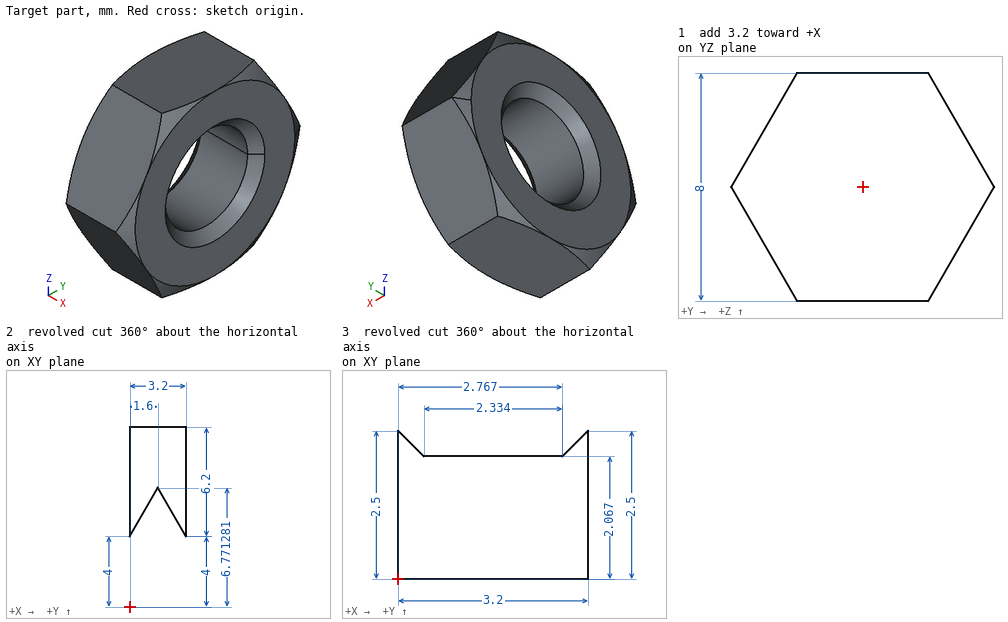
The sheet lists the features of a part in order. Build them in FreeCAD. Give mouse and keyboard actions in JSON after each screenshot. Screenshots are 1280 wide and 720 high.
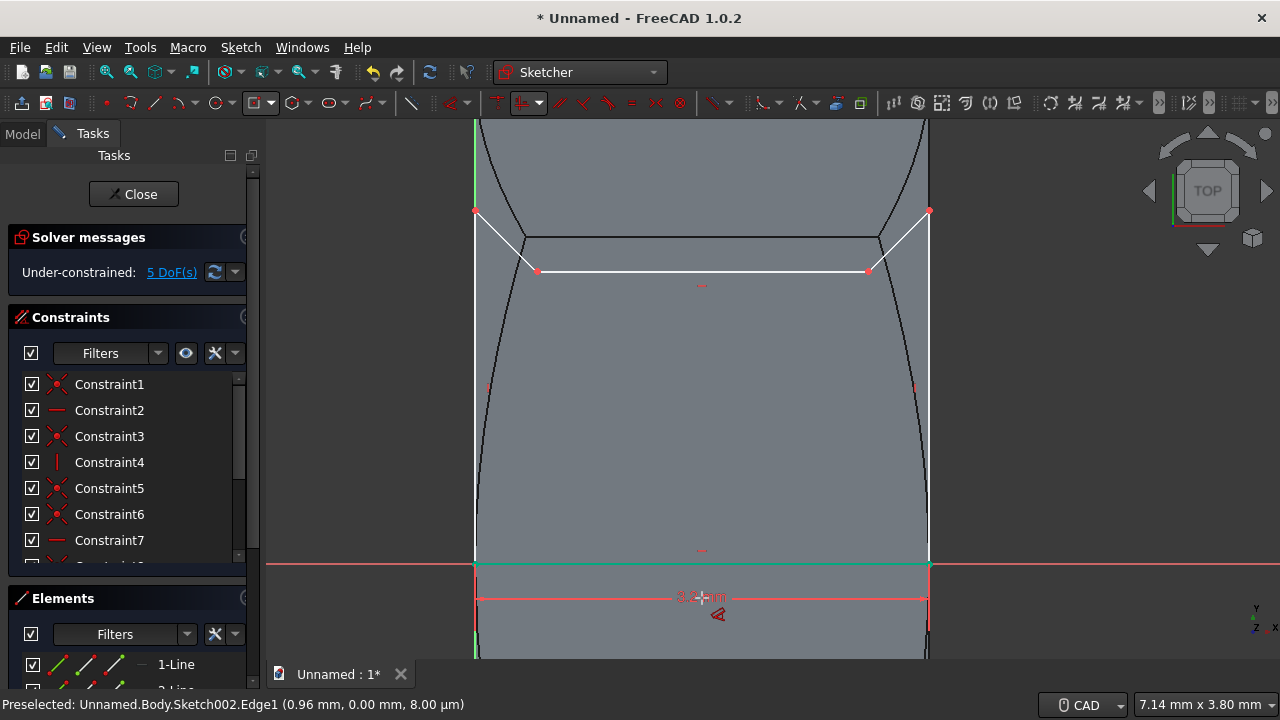
{"action": "left_click", "coordinate": [929, 458]}
{"action": "left_click", "coordinate": [963, 388]}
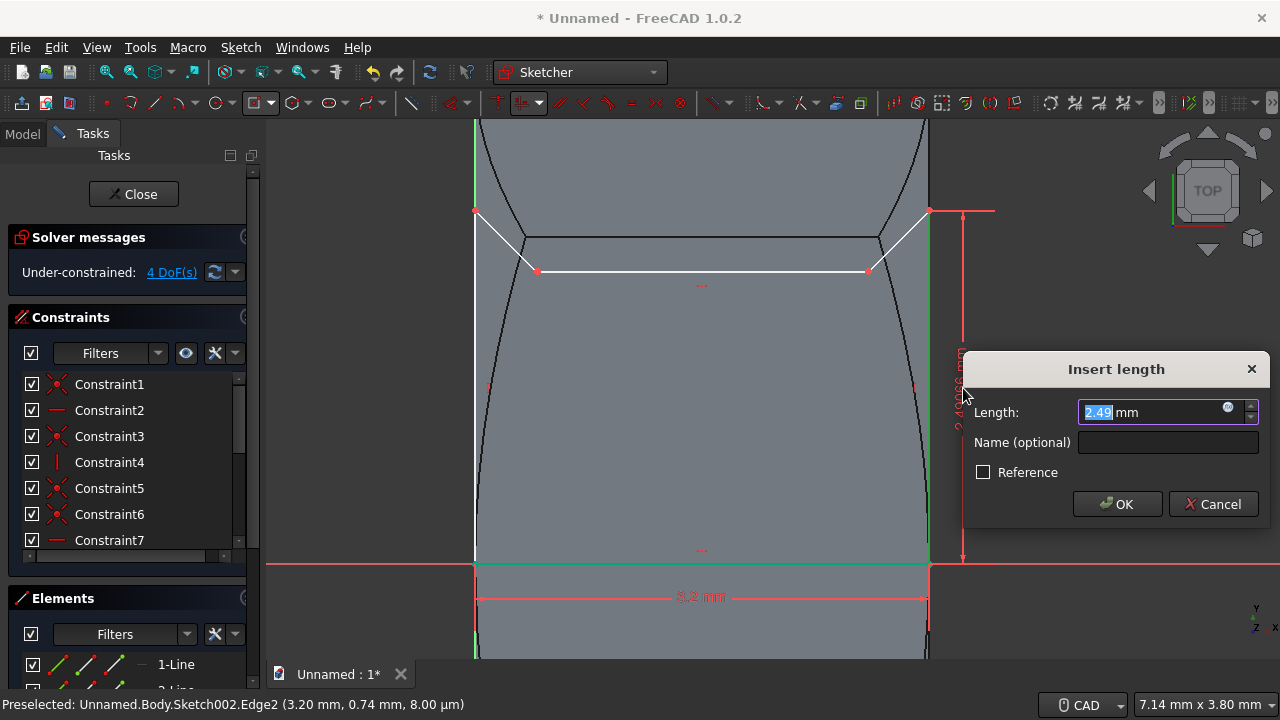
{"action": "type", "text": "2.5"}
{"action": "key", "text": "Return"}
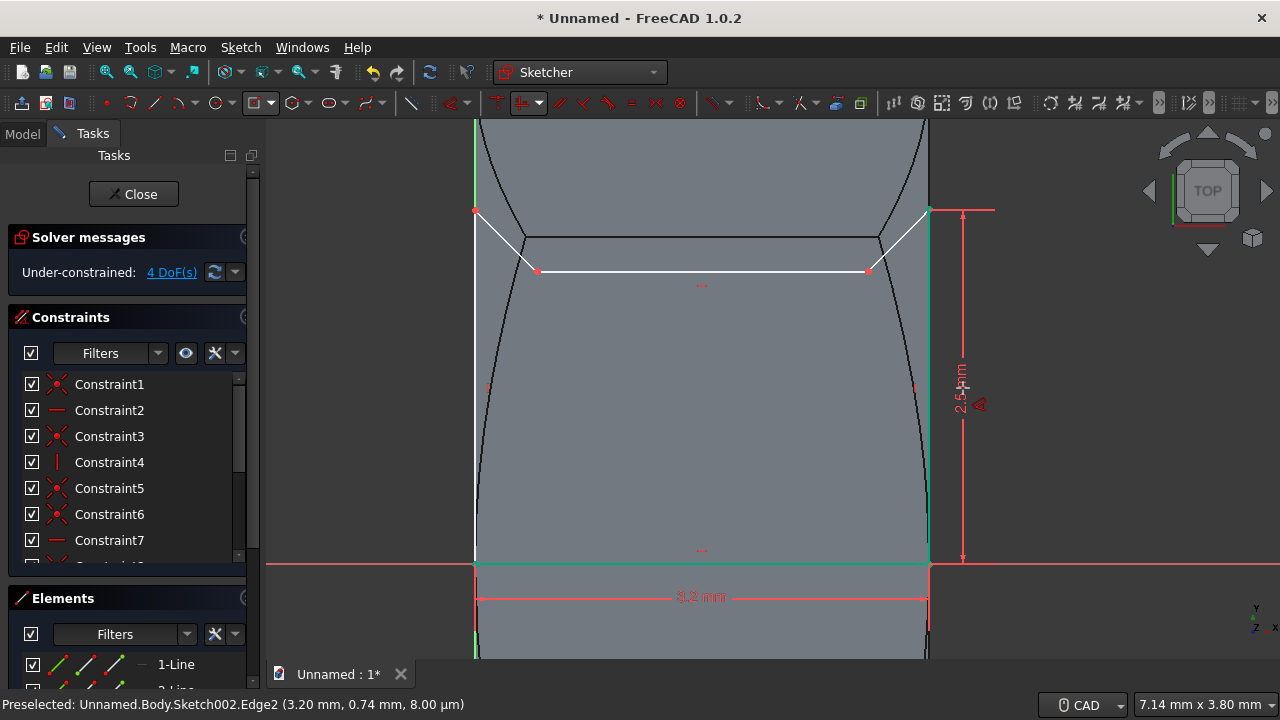
{"action": "left_click", "coordinate": [475, 317]}
{"action": "left_click", "coordinate": [441, 388]}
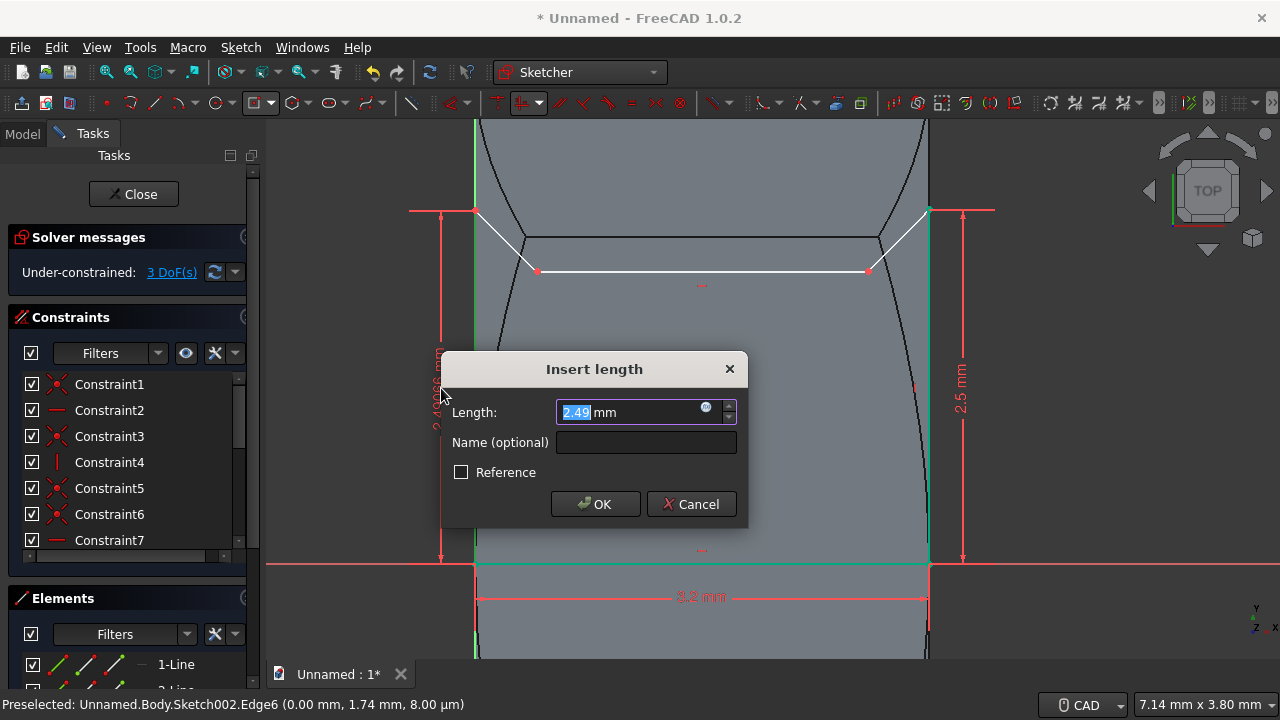
{"action": "type", "text": "2.5"}
{"action": "key", "text": "Return"}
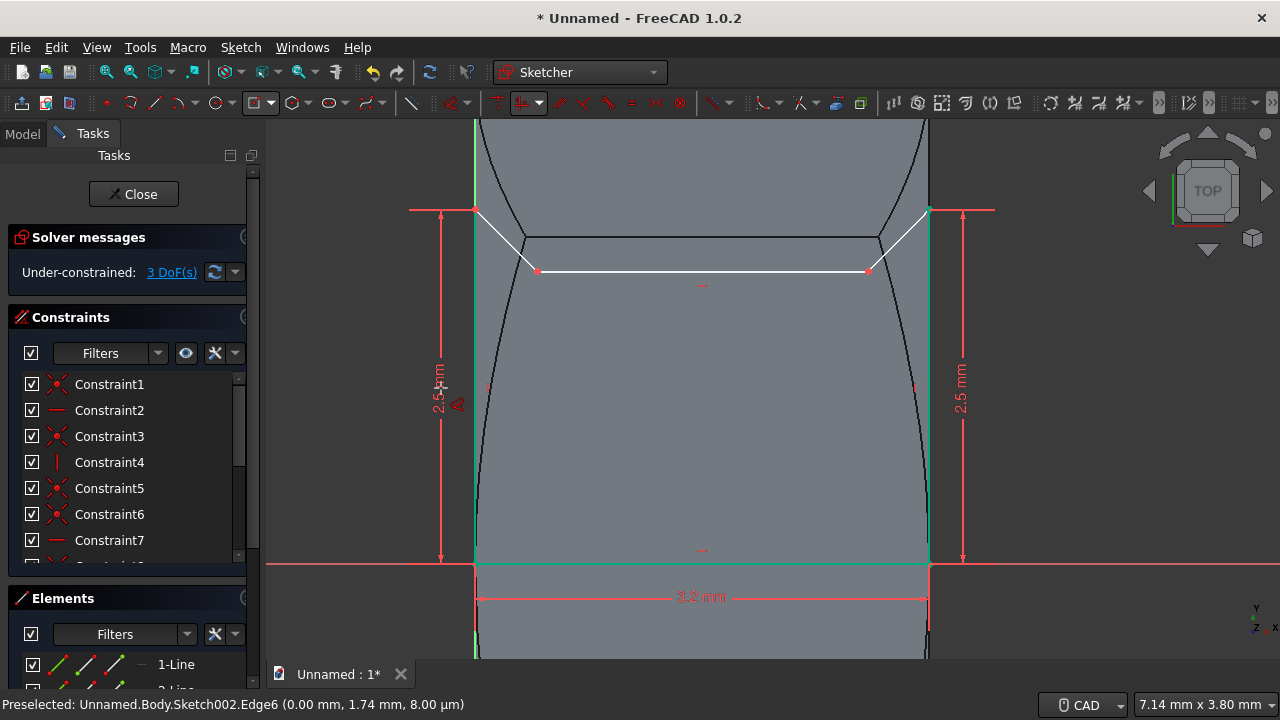
{"action": "left_click", "coordinate": [769, 272]}
{"action": "left_click", "coordinate": [702, 238]}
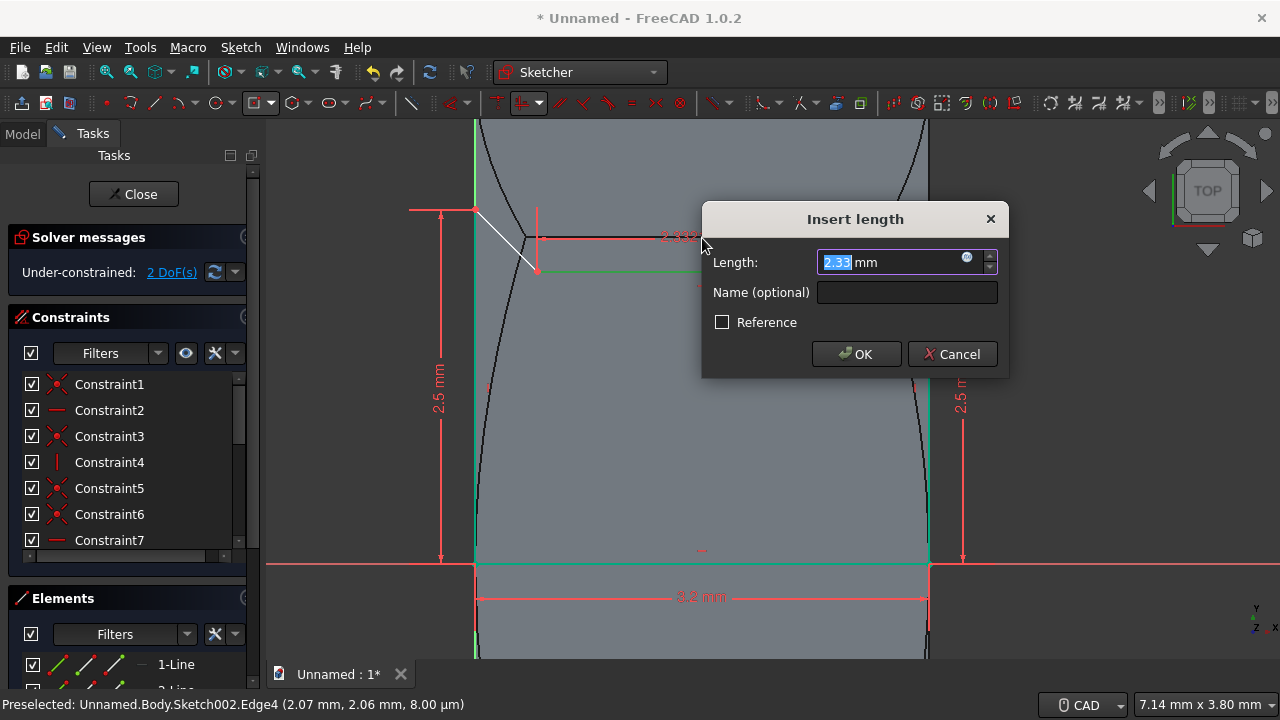
{"action": "type", "text": "2.334"}
{"action": "key", "text": "Return"}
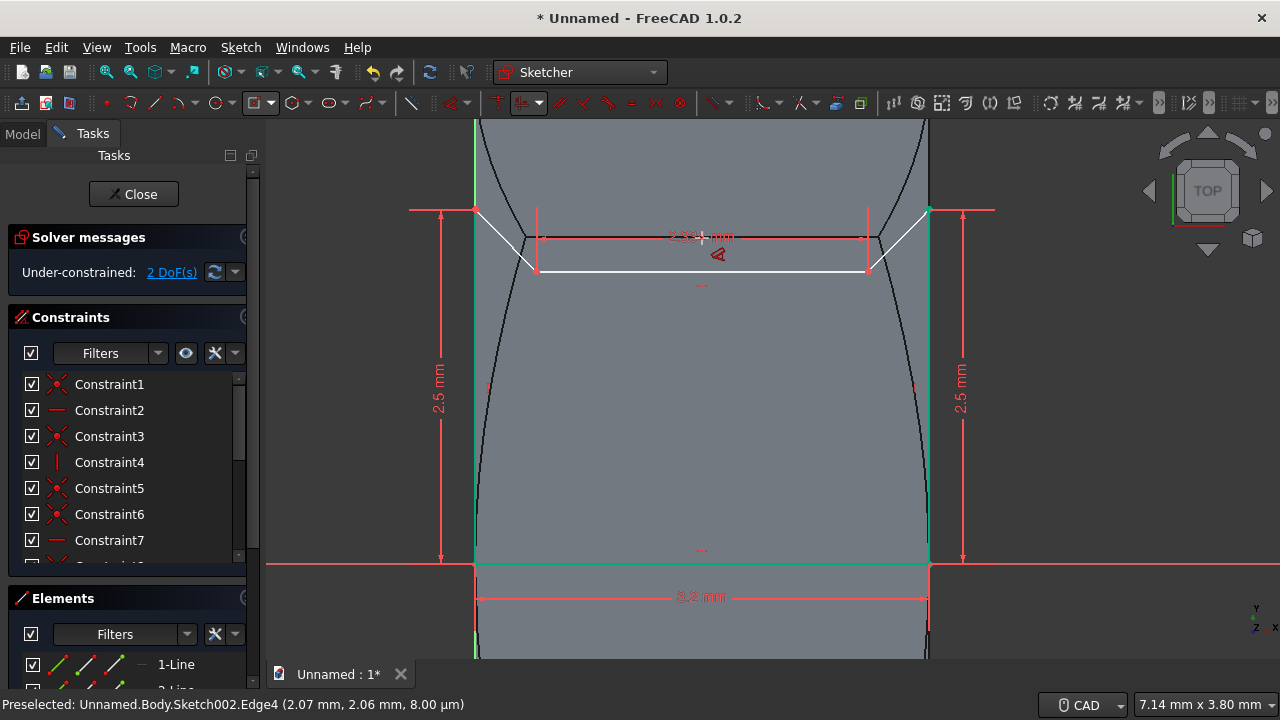
{"action": "left_click", "coordinate": [868, 272]}
{"action": "left_click", "coordinate": [581, 598]}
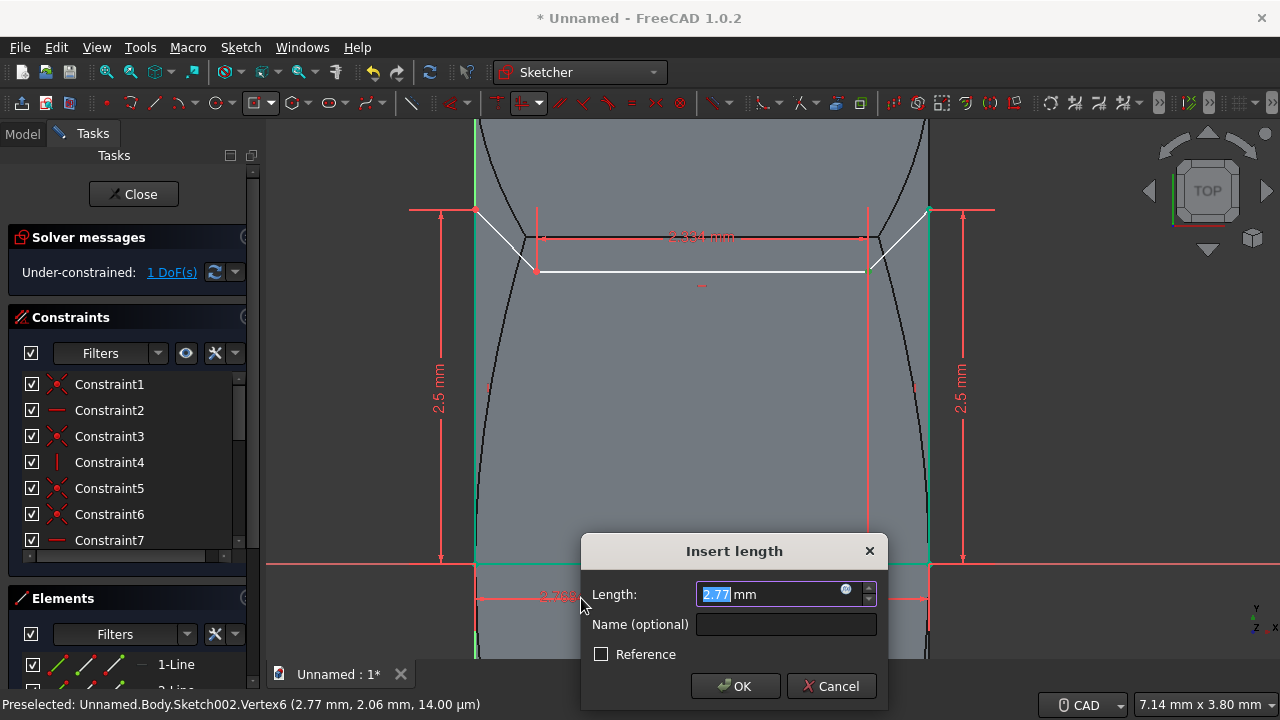
{"action": "type", "text": "2.767"}
{"action": "key", "text": "Return"}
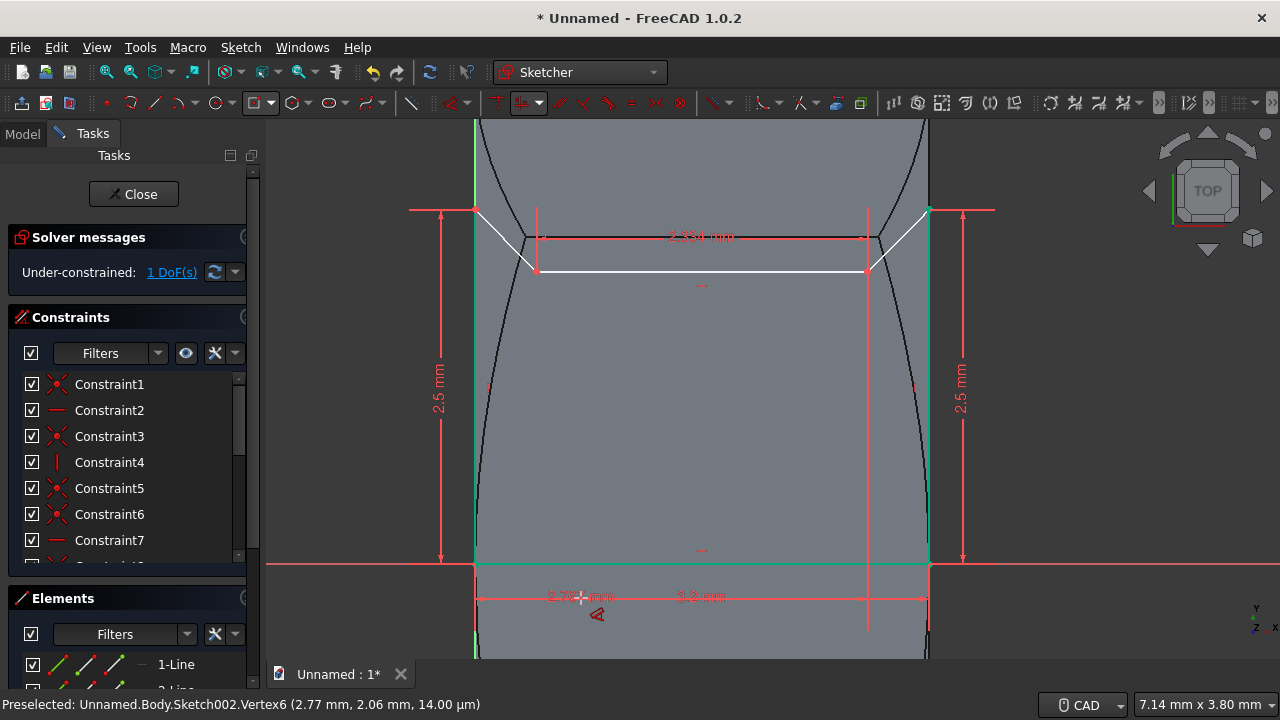
{"action": "left_click", "coordinate": [868, 272]}
{"action": "left_click", "coordinate": [441, 418]}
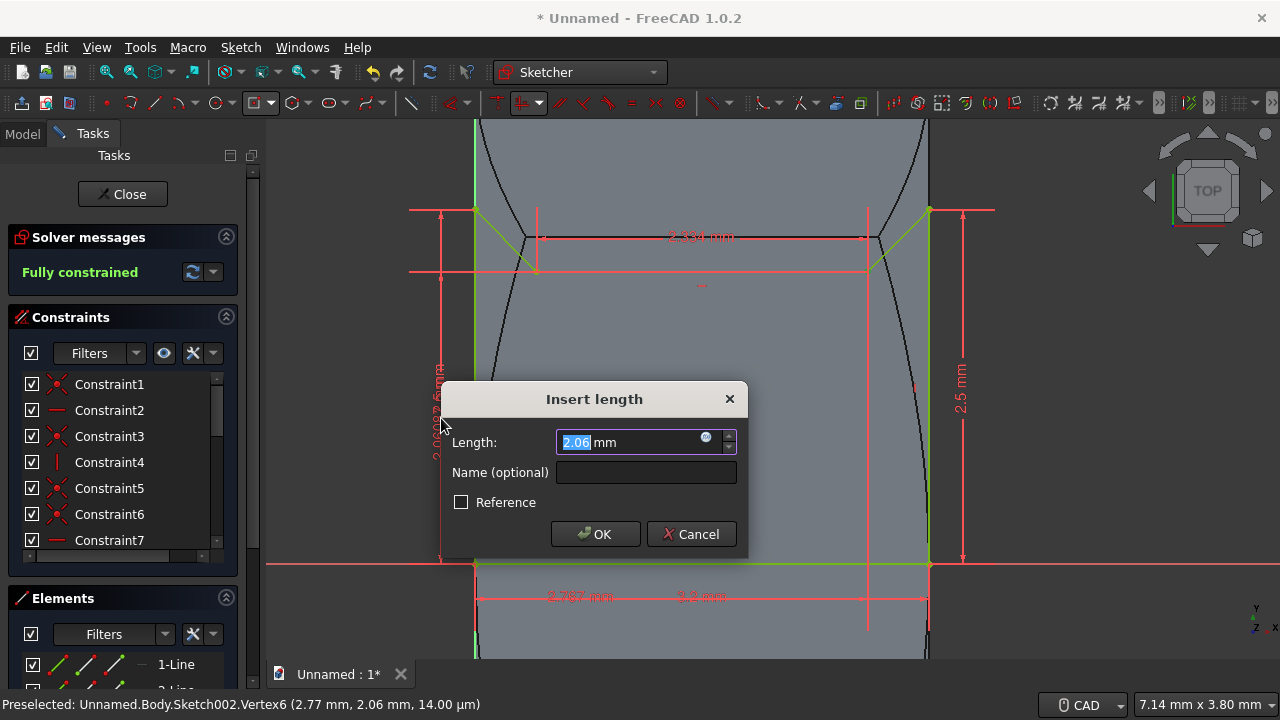
{"action": "type", "text": "2.067"}
{"action": "key", "text": "Return"}
{"action": "key", "text": "Escape"}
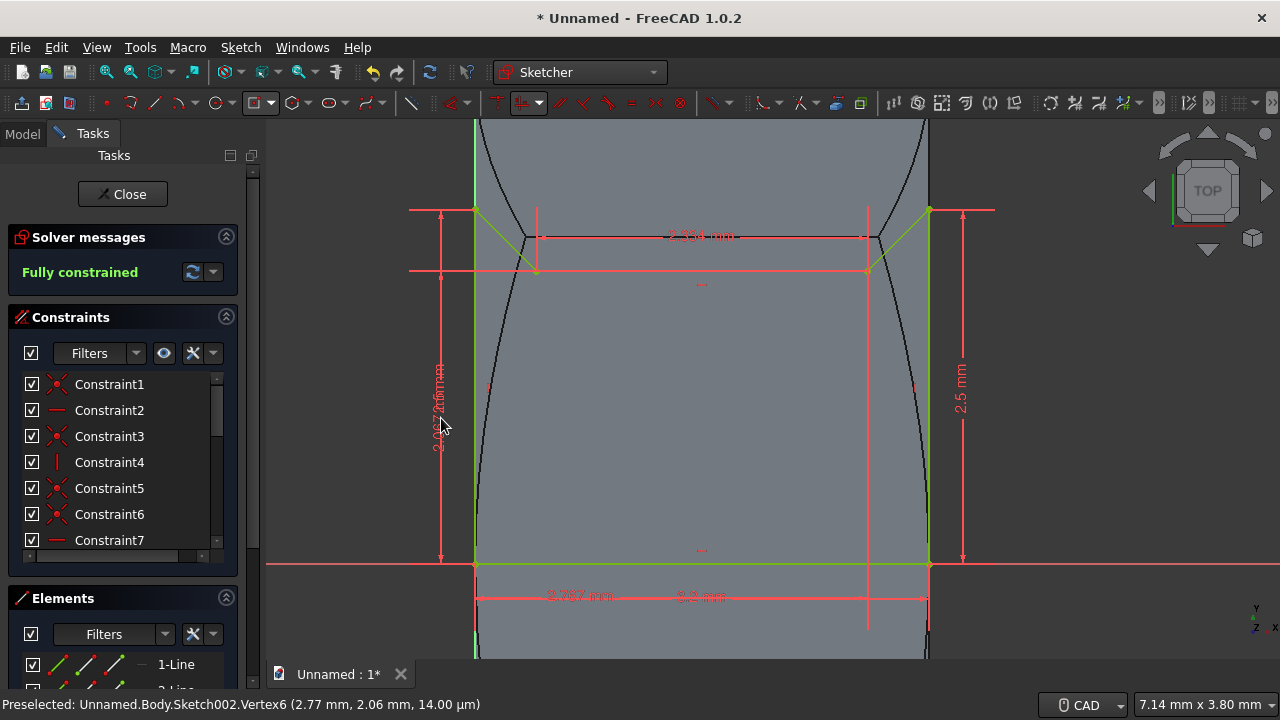
{"action": "left_click", "coordinate": [123, 194]}